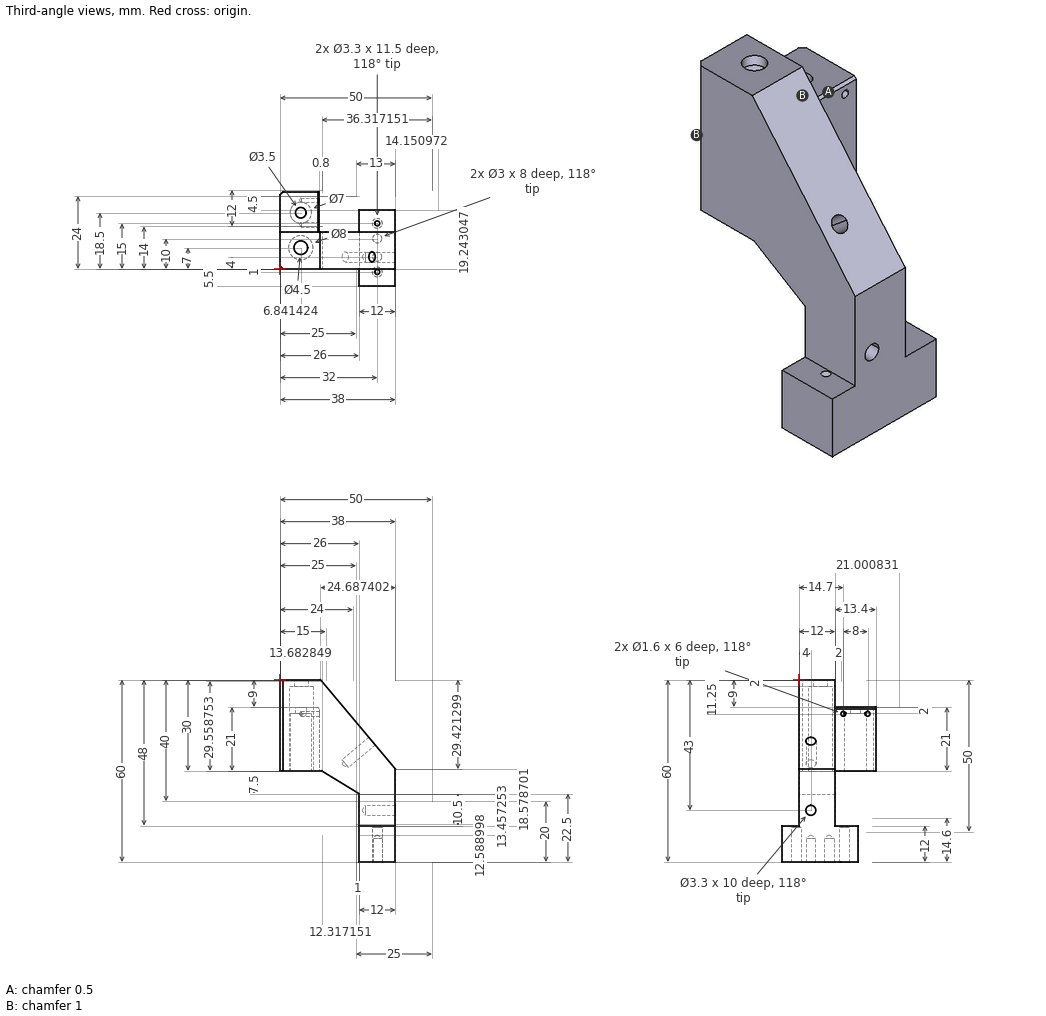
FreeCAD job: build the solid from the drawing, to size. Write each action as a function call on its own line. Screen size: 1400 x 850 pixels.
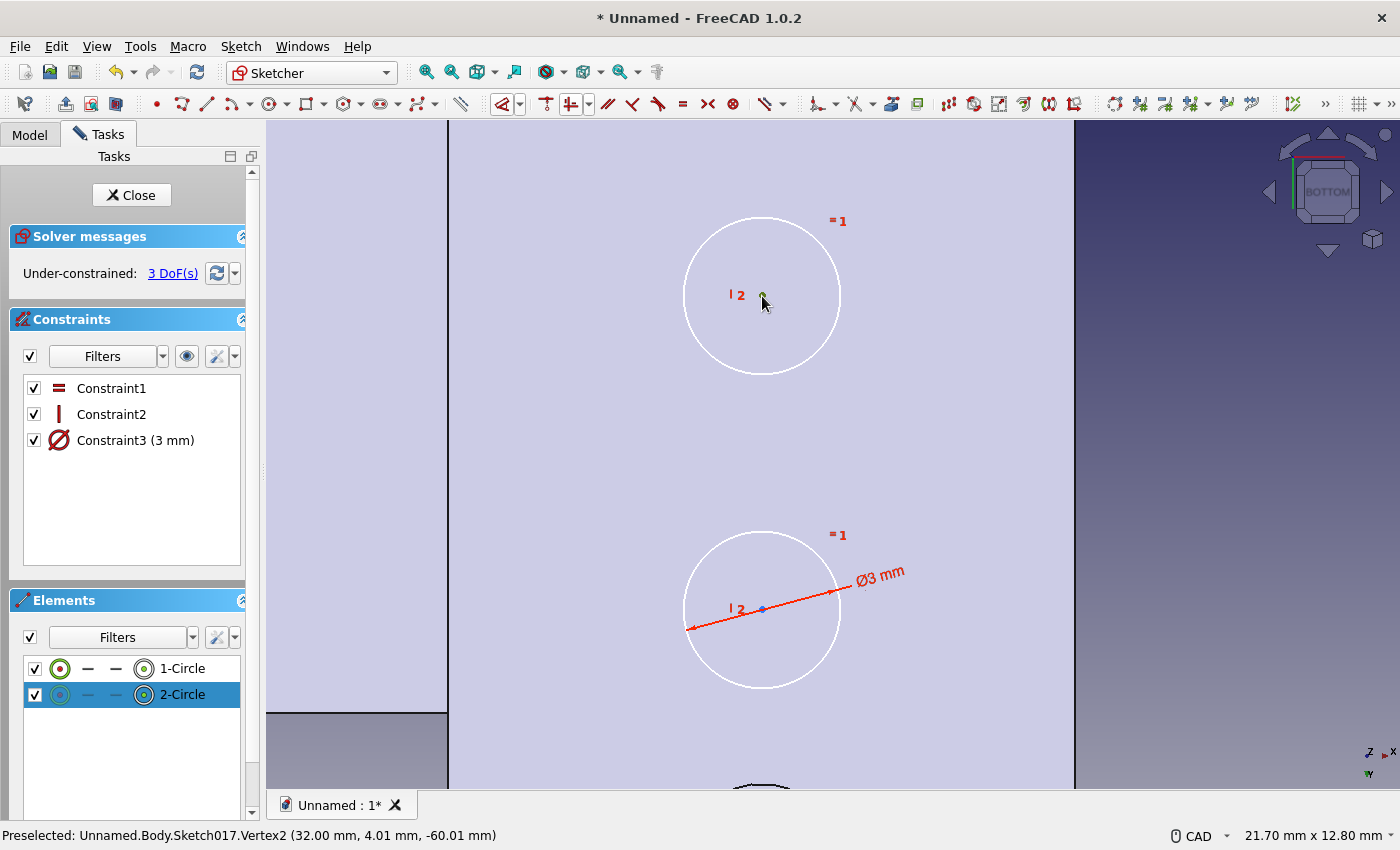
key(i)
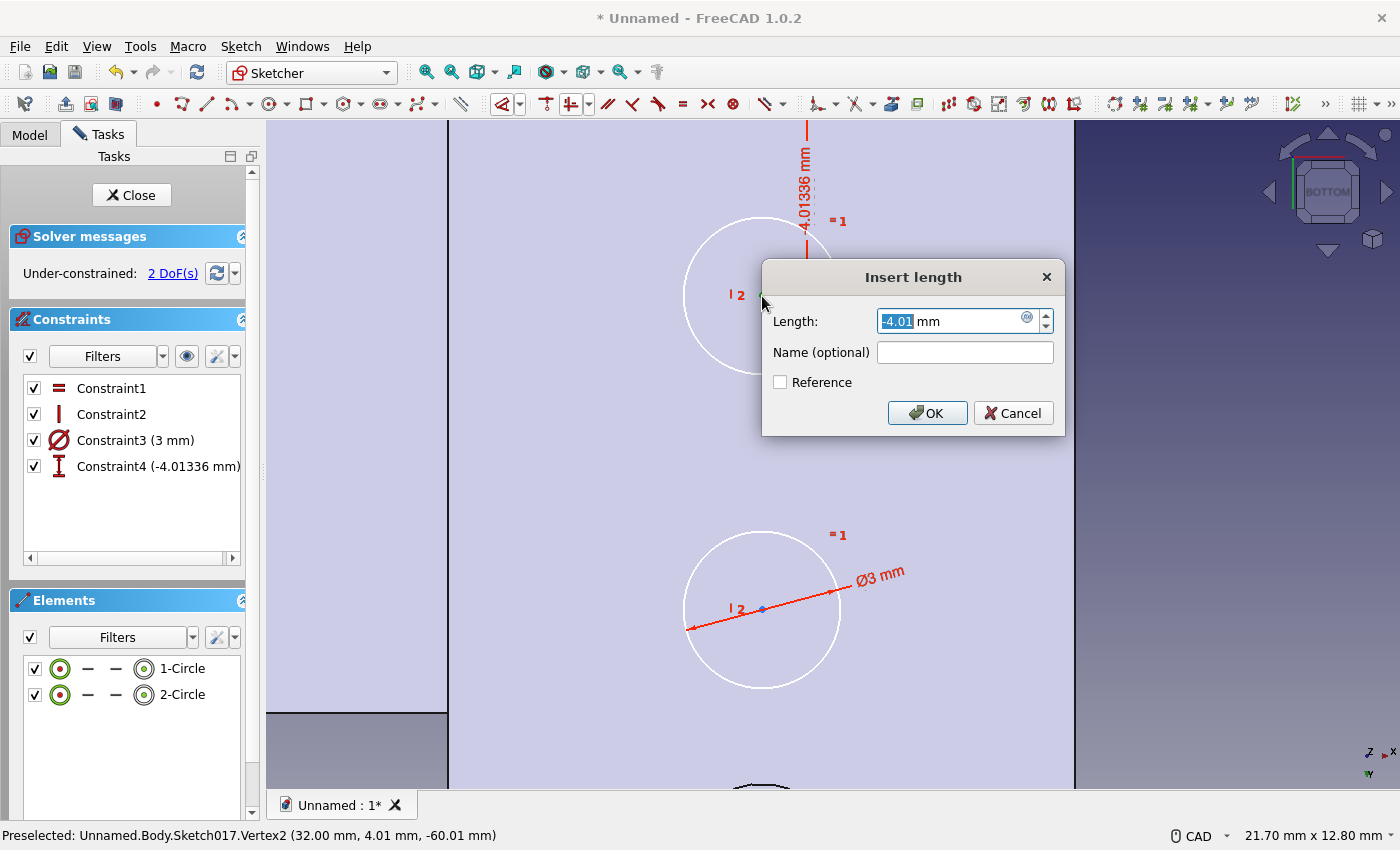
text(-4)
key(Return)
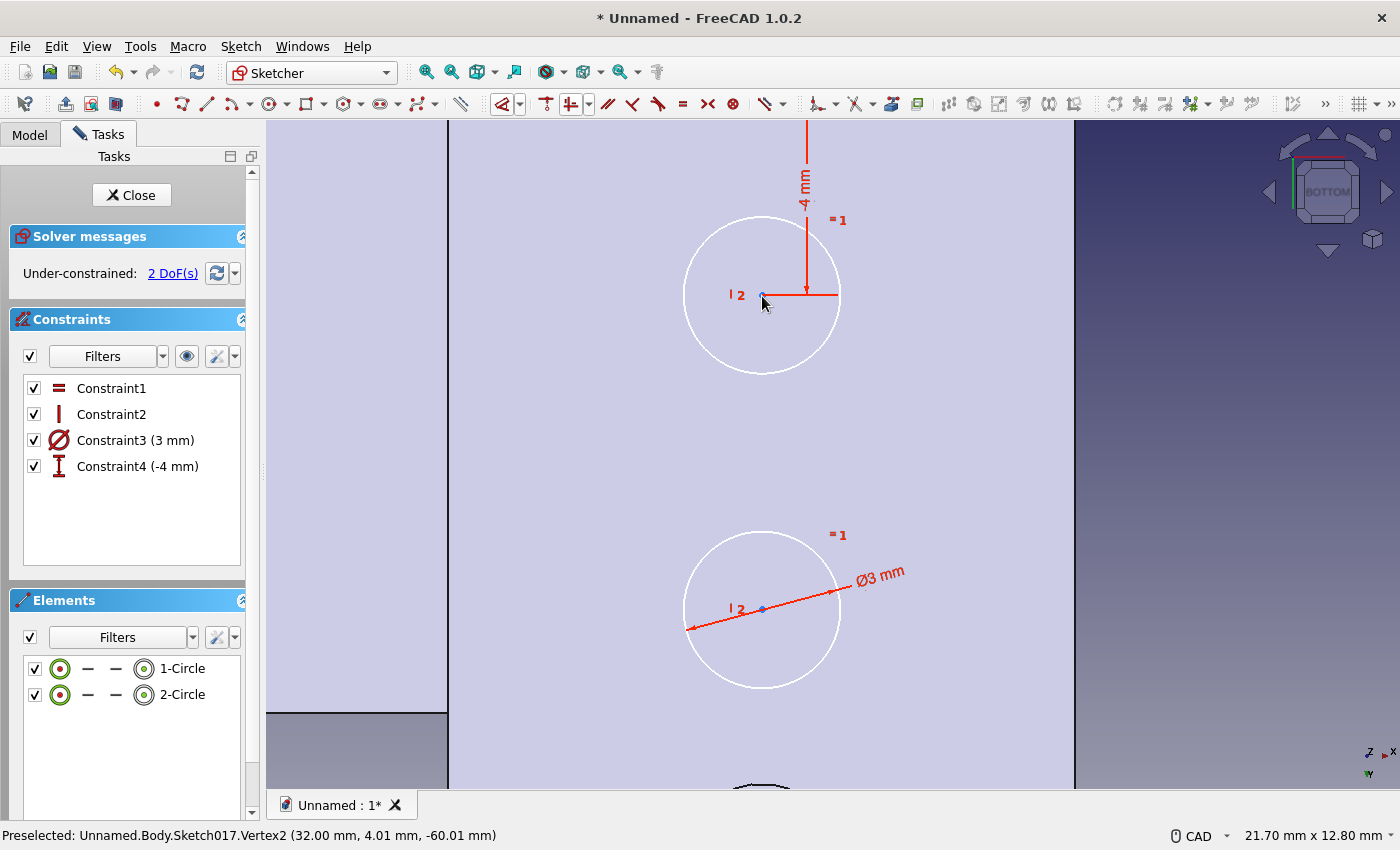
click(762, 610)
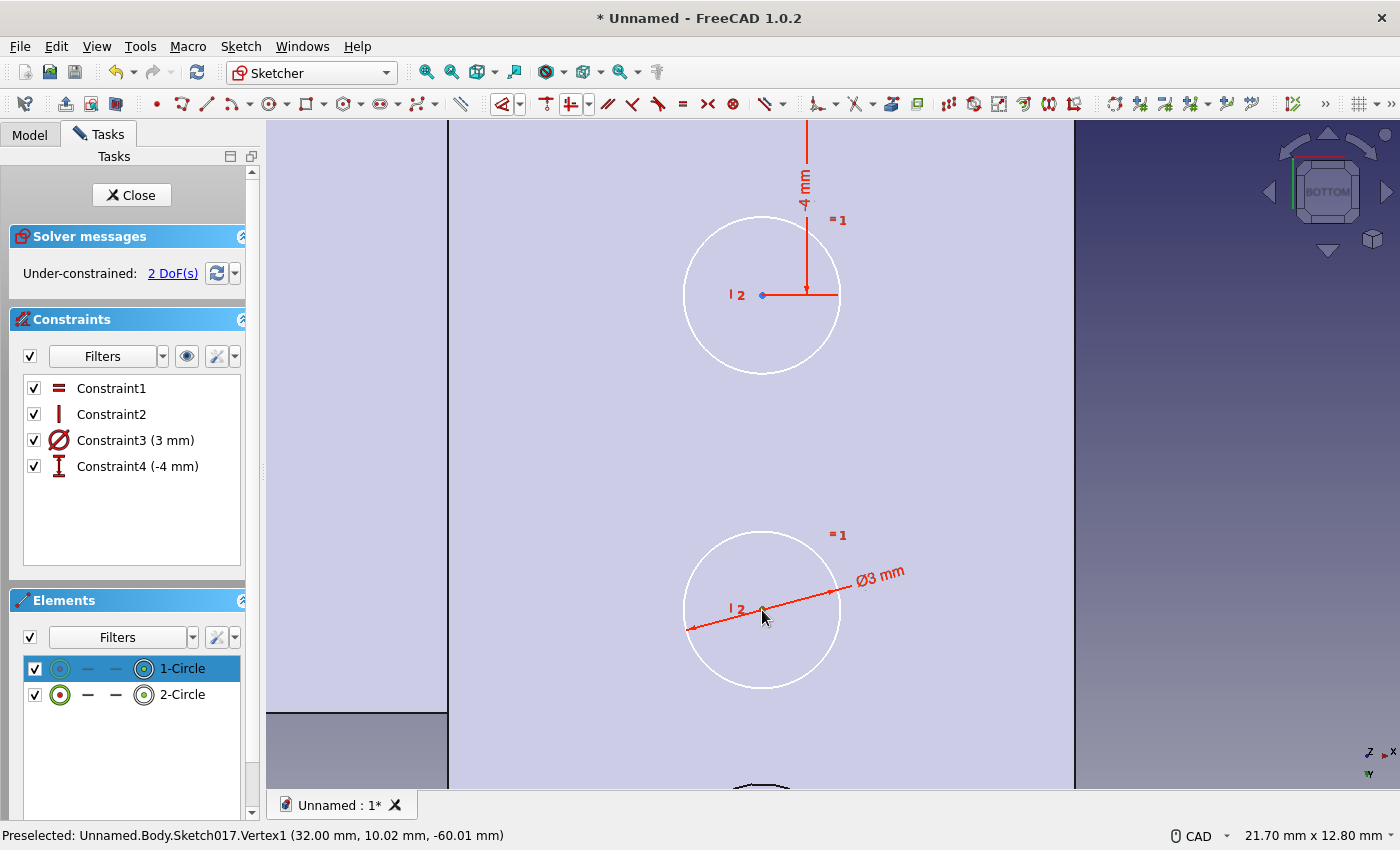
key(l)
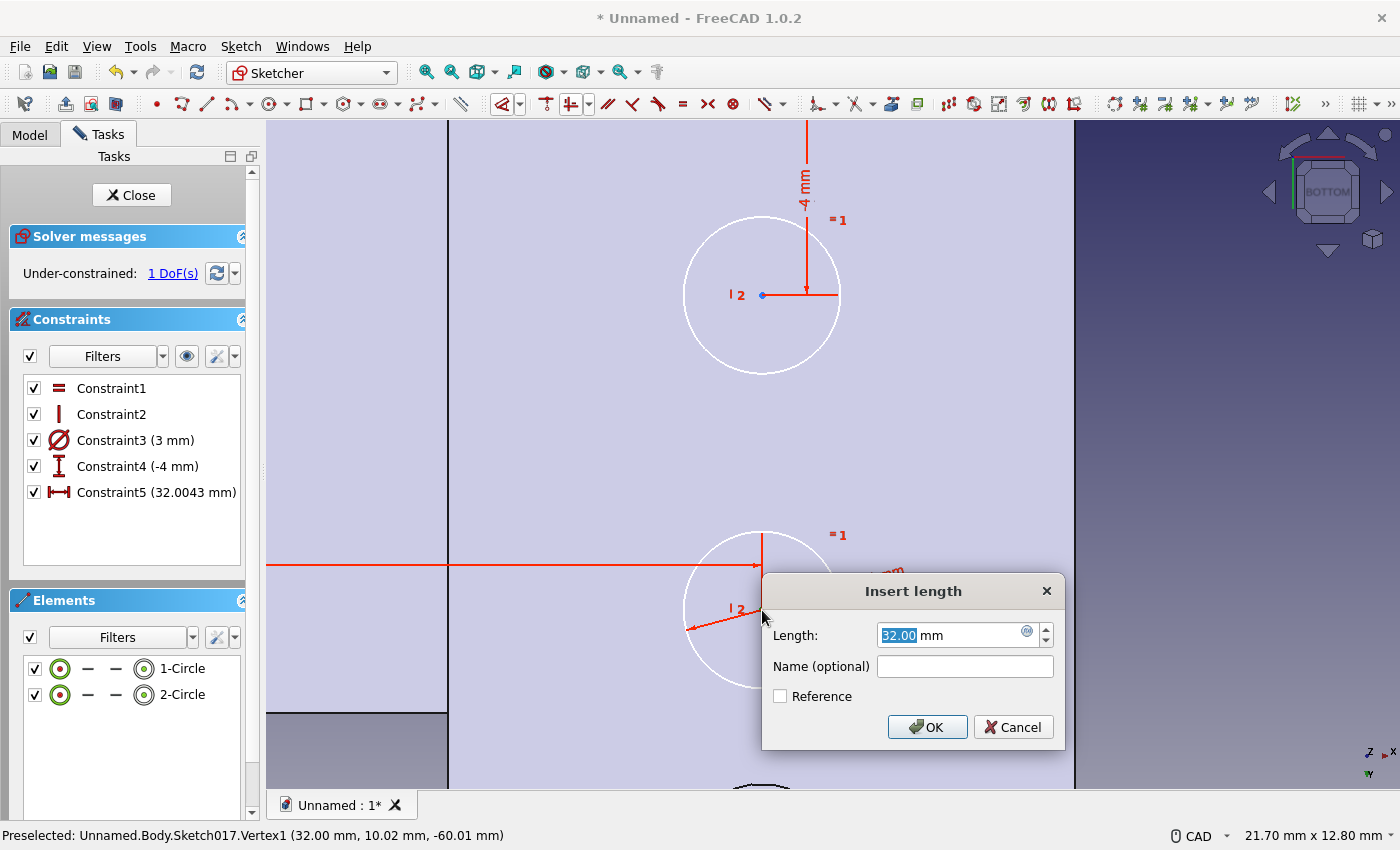
text(32)
key(Return)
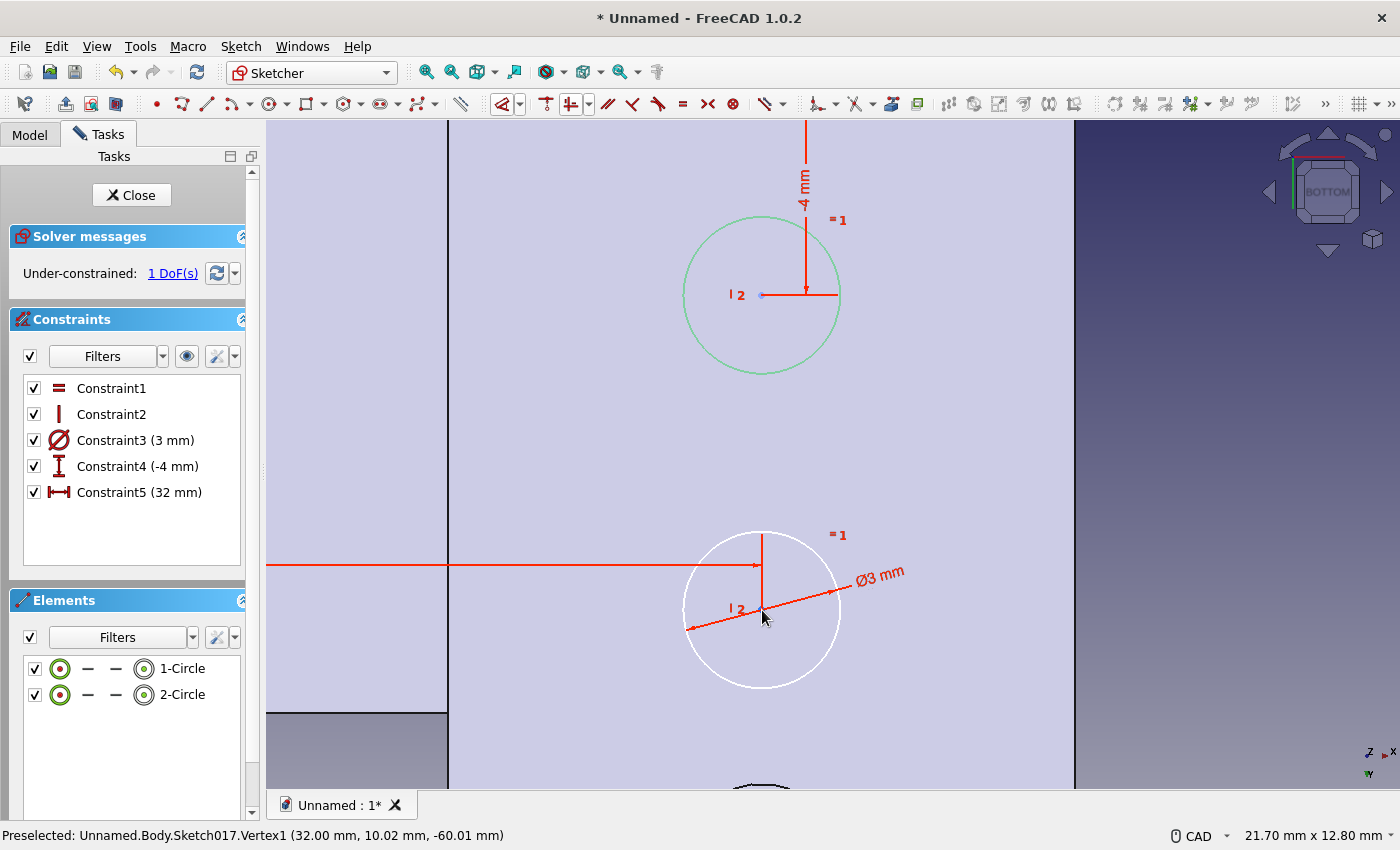
click(762, 610)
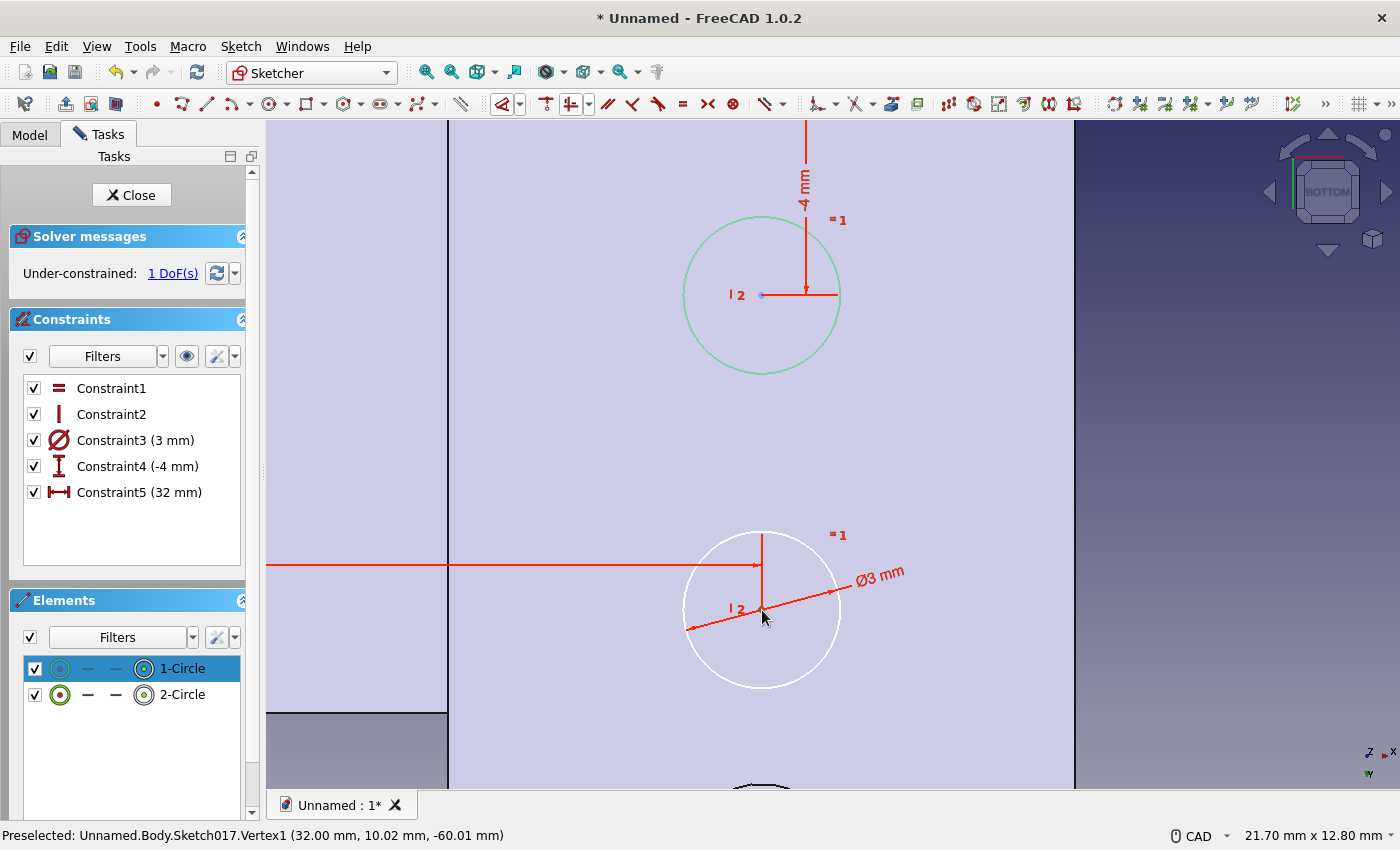
key(i)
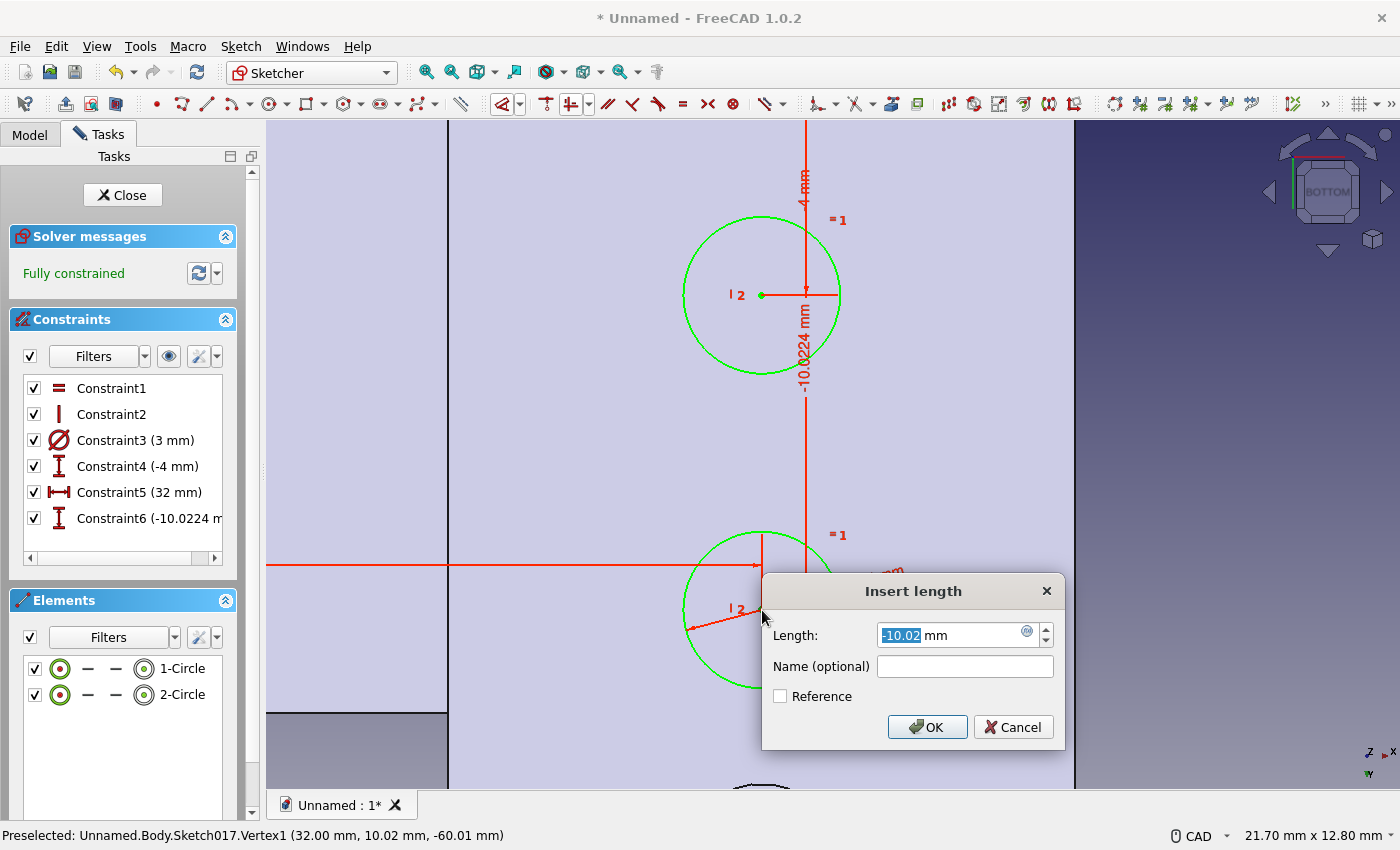
text(-10)
key(Return)